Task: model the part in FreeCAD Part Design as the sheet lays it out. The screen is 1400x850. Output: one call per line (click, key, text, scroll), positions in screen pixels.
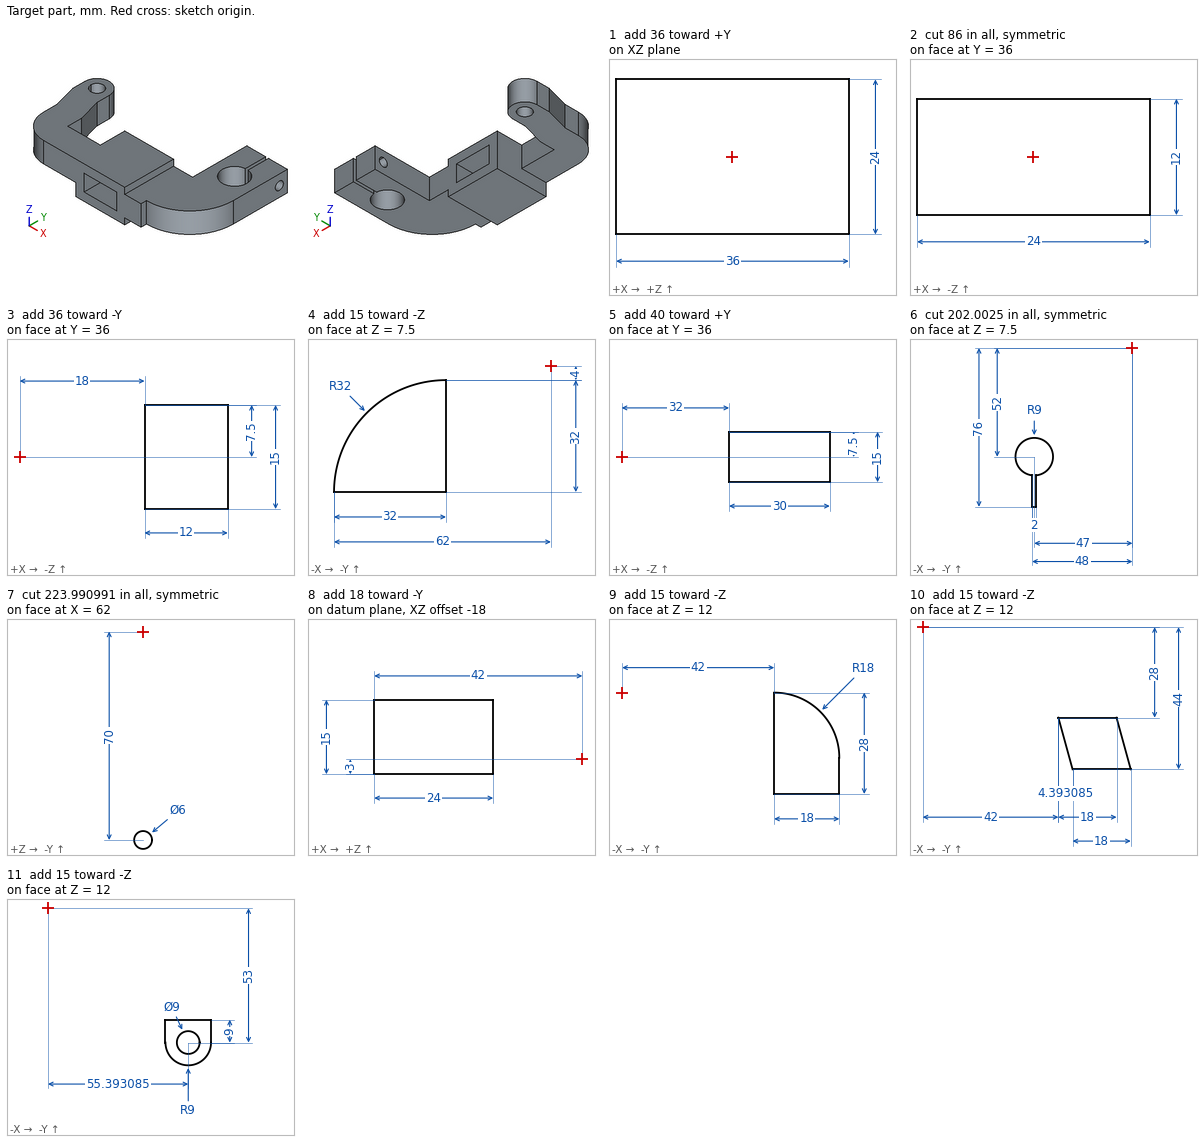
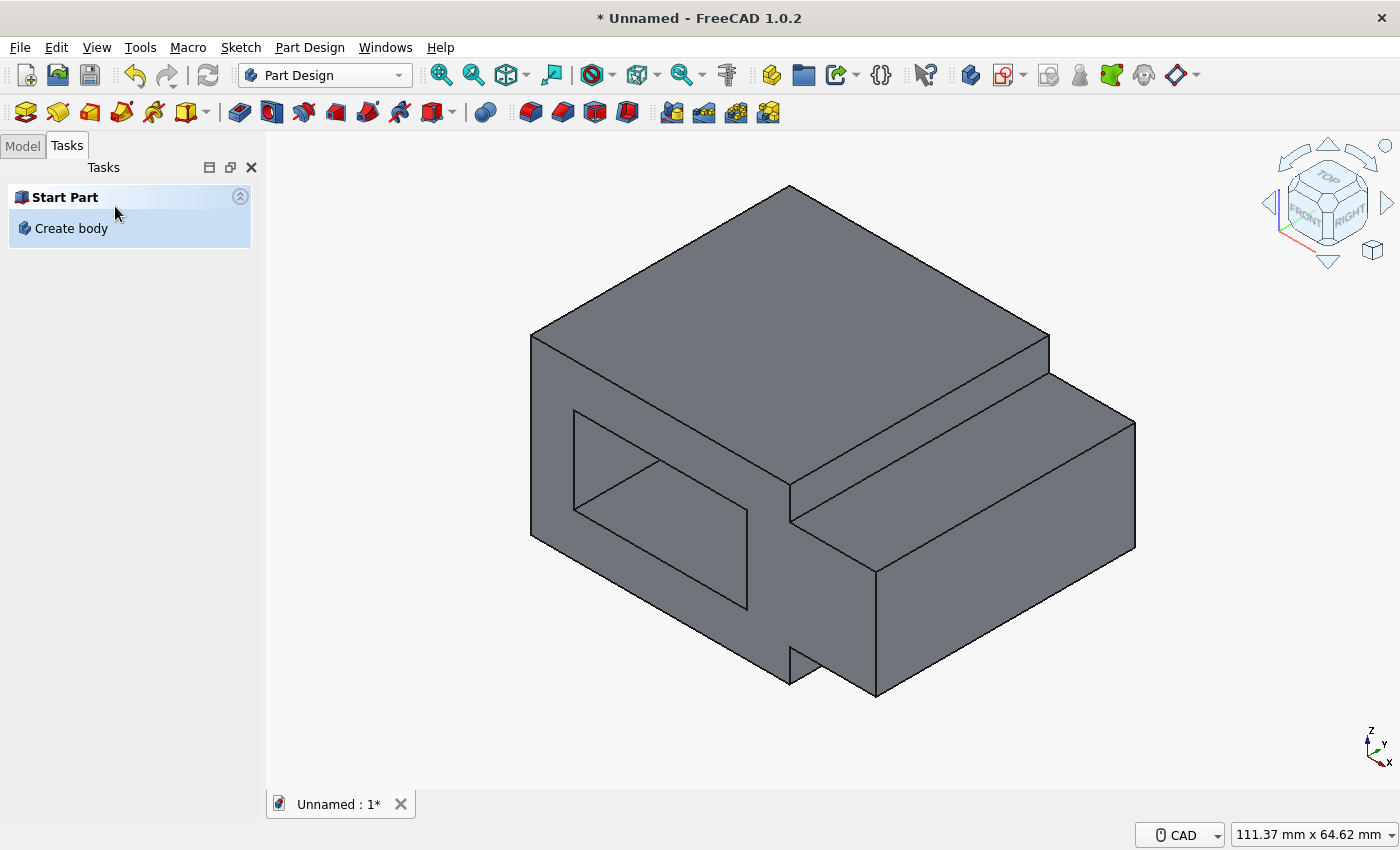
click(1037, 429)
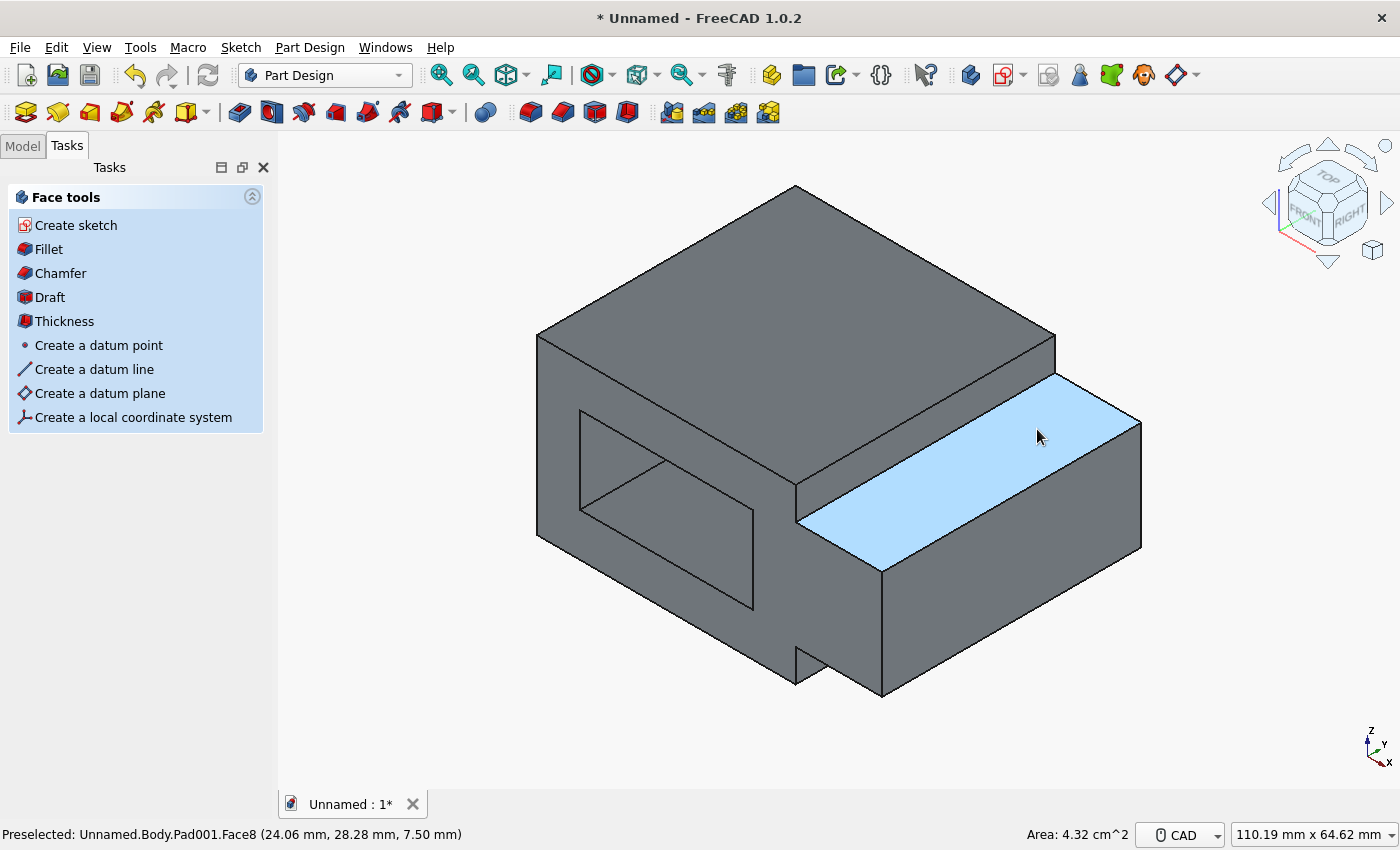
click(1004, 76)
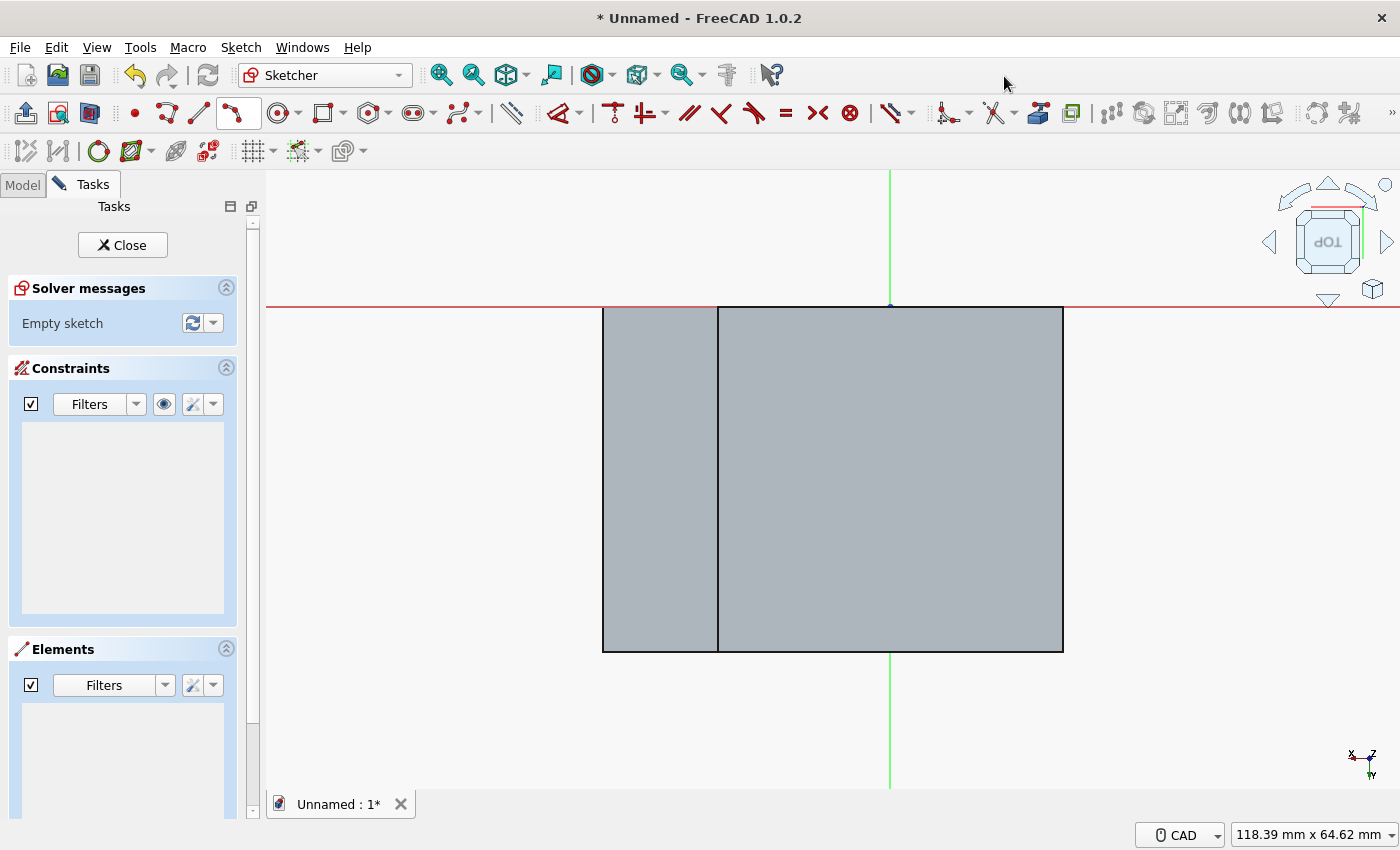
scroll(1235, 480, down, 1)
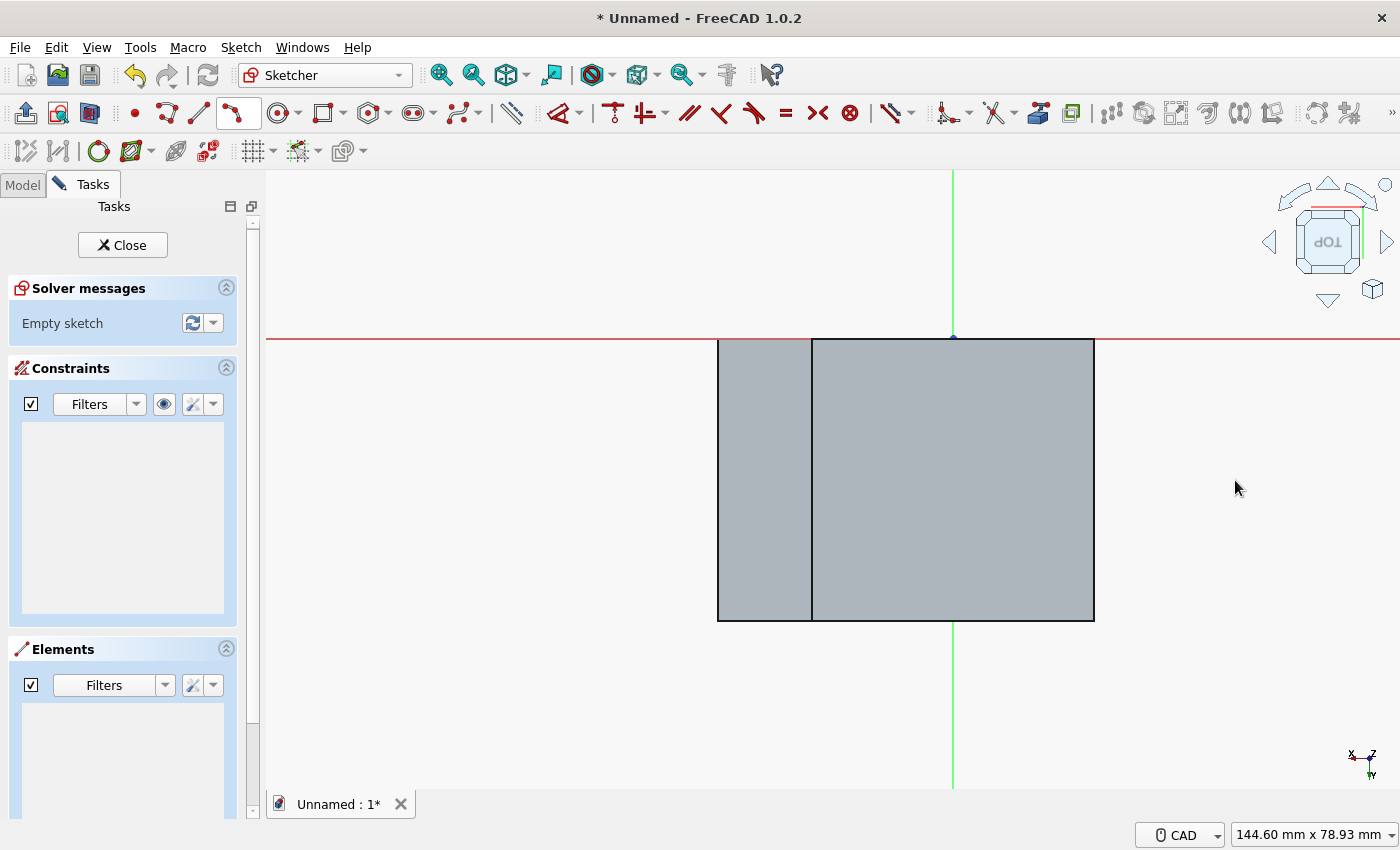
scroll(599, 480, up, 2)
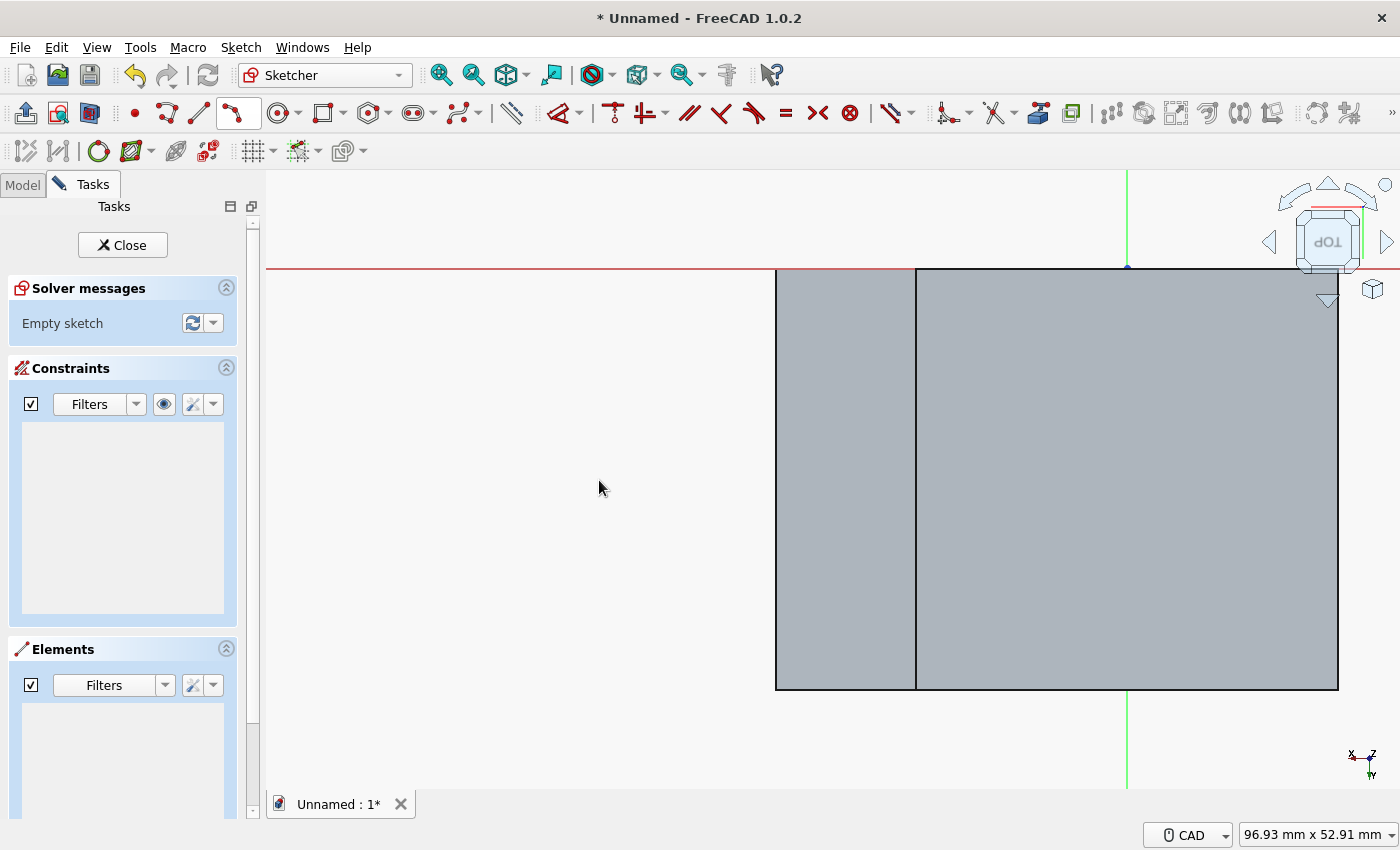
key(g)
key(m)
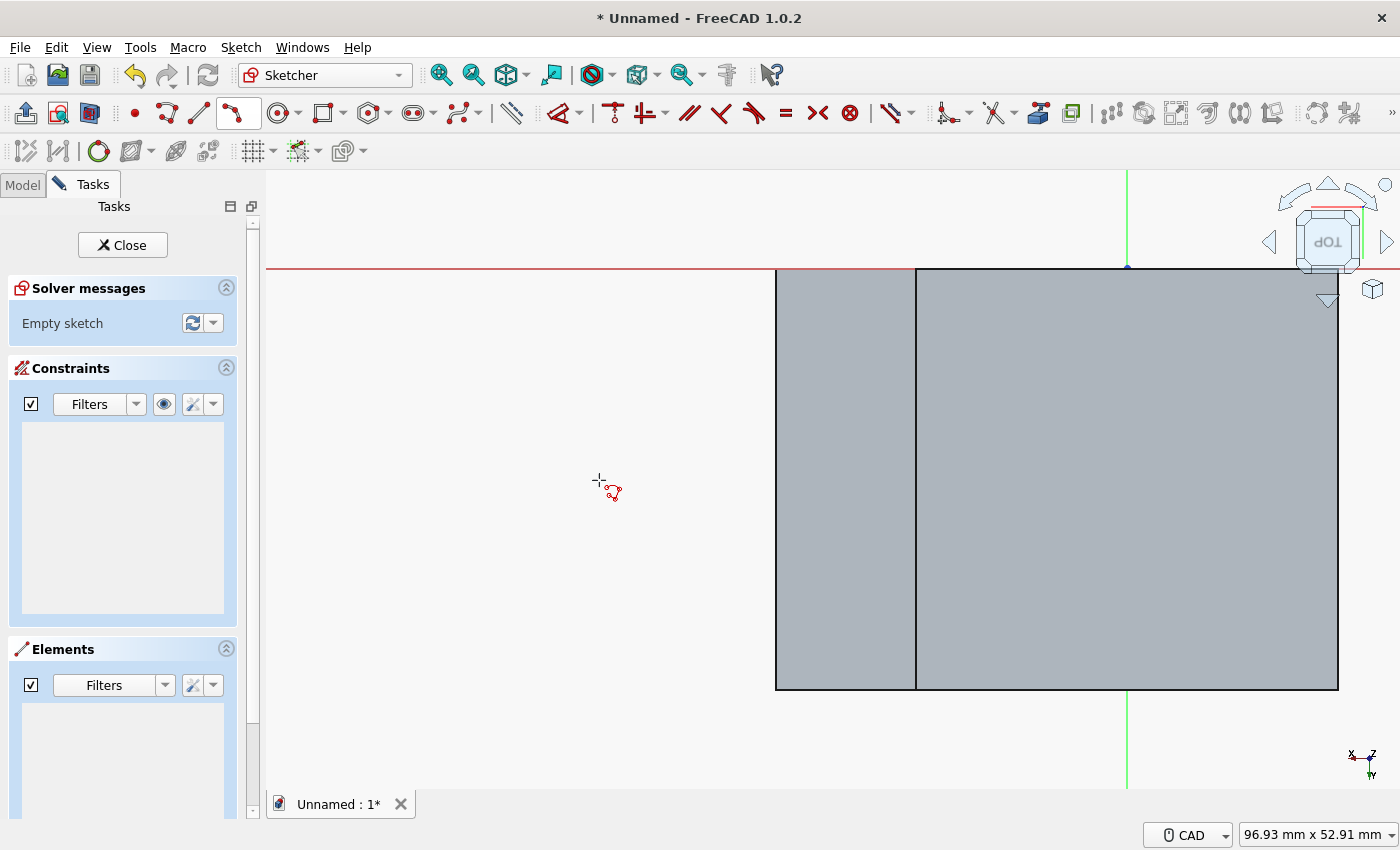
click(402, 690)
click(776, 690)
click(776, 315)
right_click(776, 315)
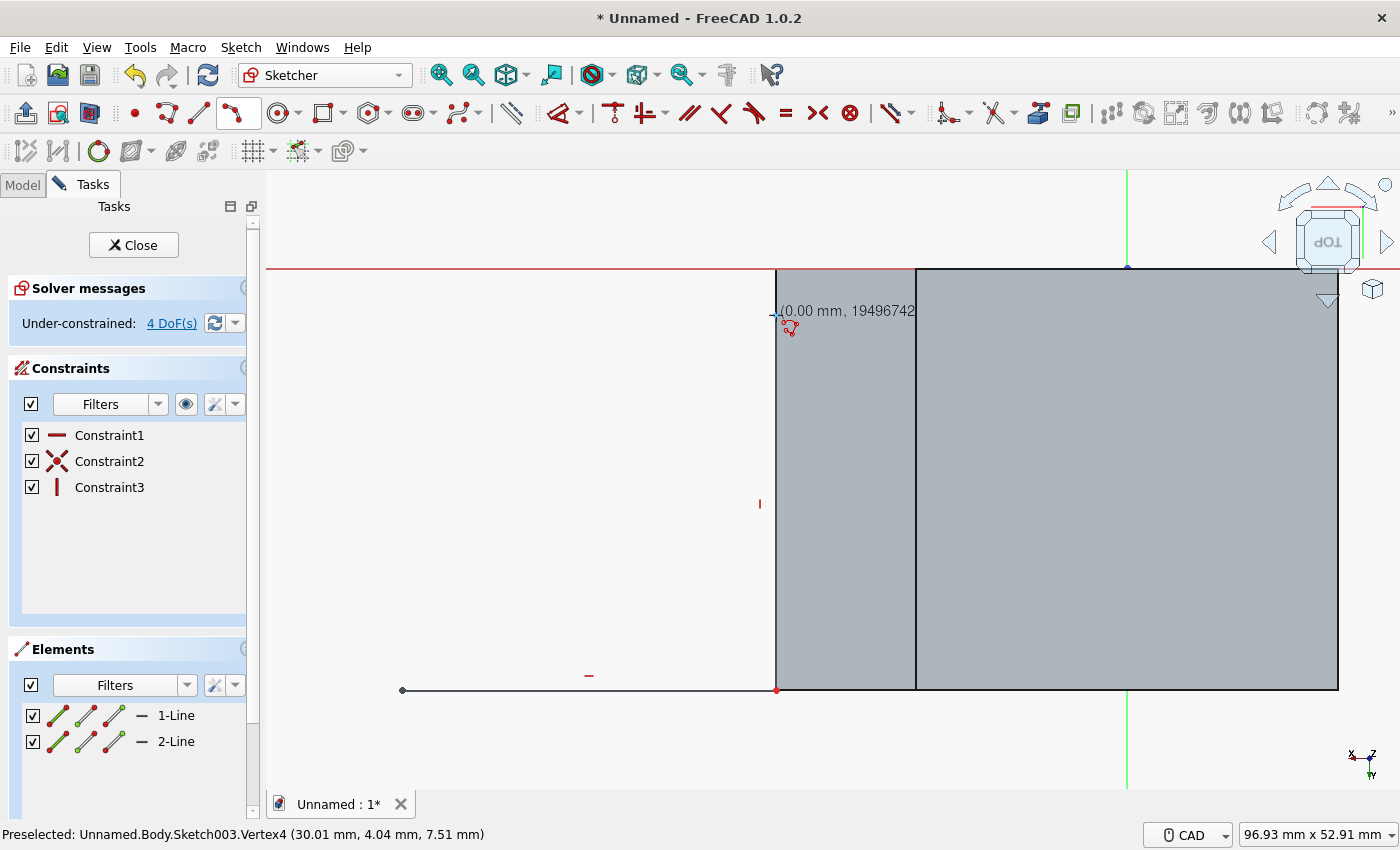
key(g)
key(3)
key(a)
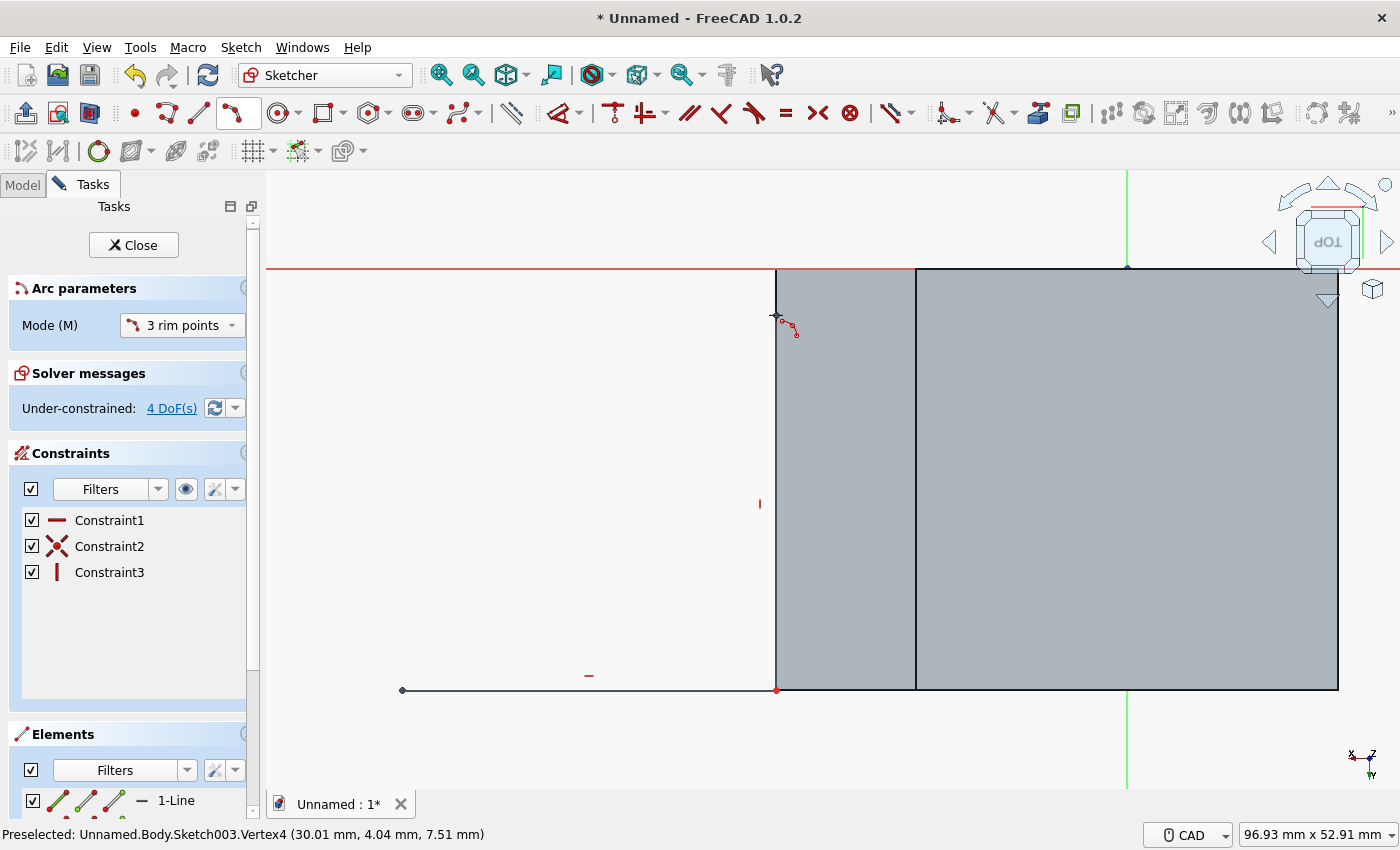
click(776, 316)
click(402, 691)
click(511, 425)
key(Escape)